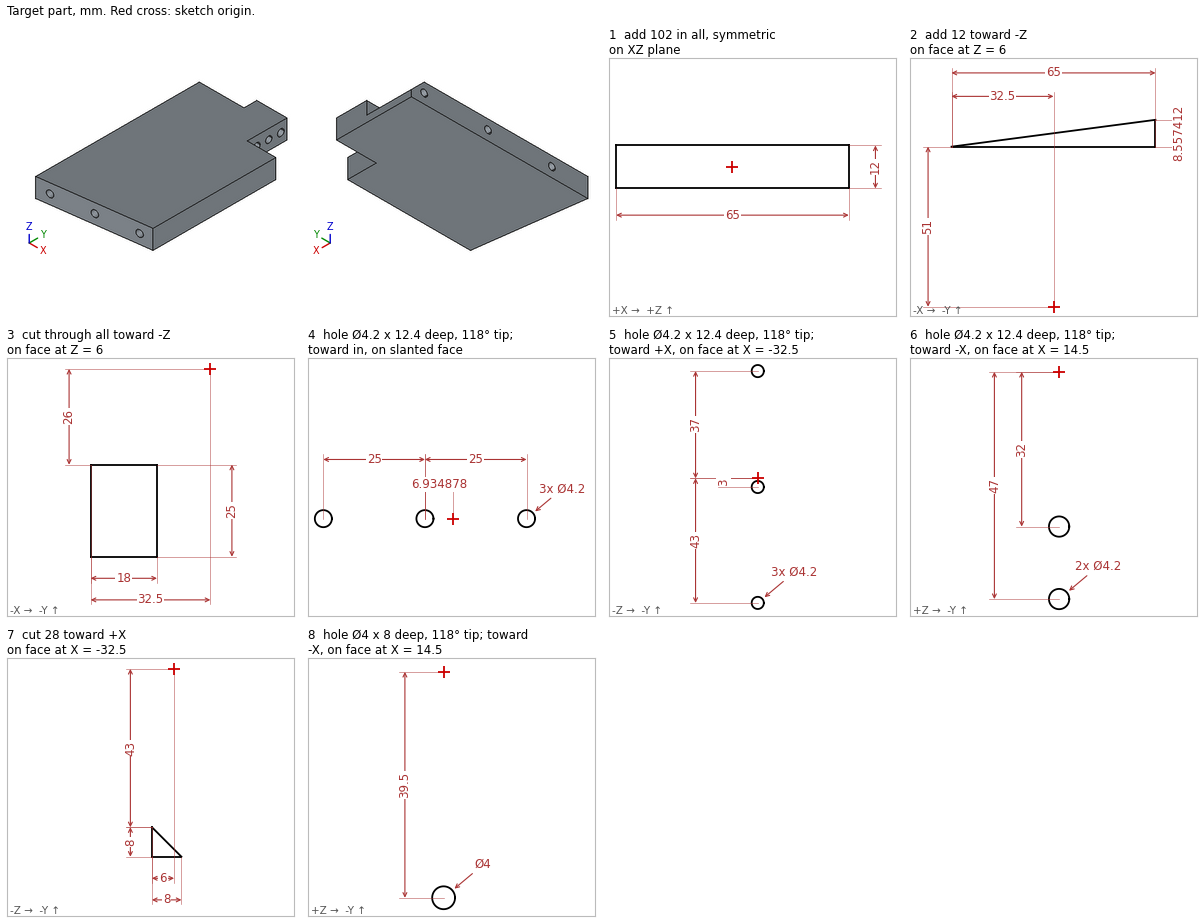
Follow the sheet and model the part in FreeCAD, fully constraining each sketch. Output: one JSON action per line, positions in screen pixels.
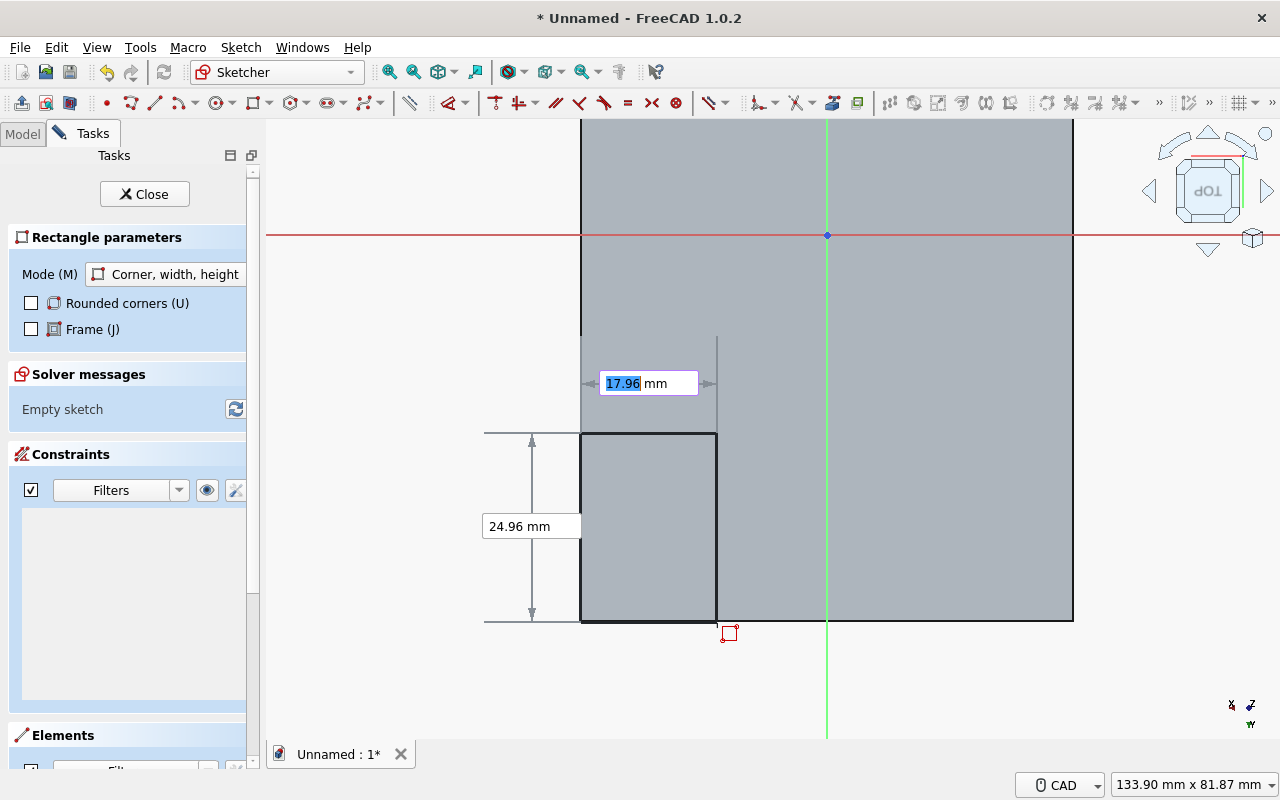
{"action": "type", "text": "18"}
{"action": "key", "text": "Tab"}
{"action": "type", "text": "25"}
{"action": "key", "text": "Return"}
{"action": "key", "text": "Escape"}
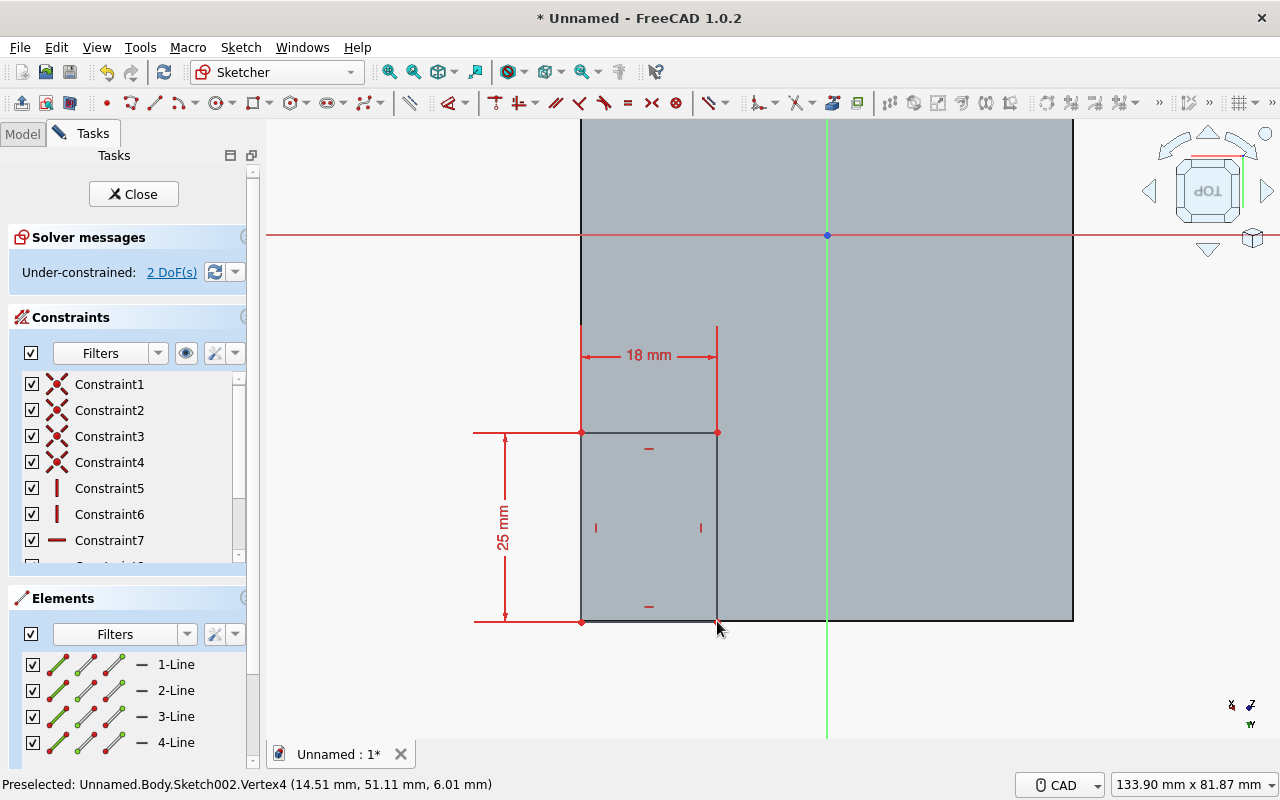
{"action": "left_click", "coordinate": [448, 104]}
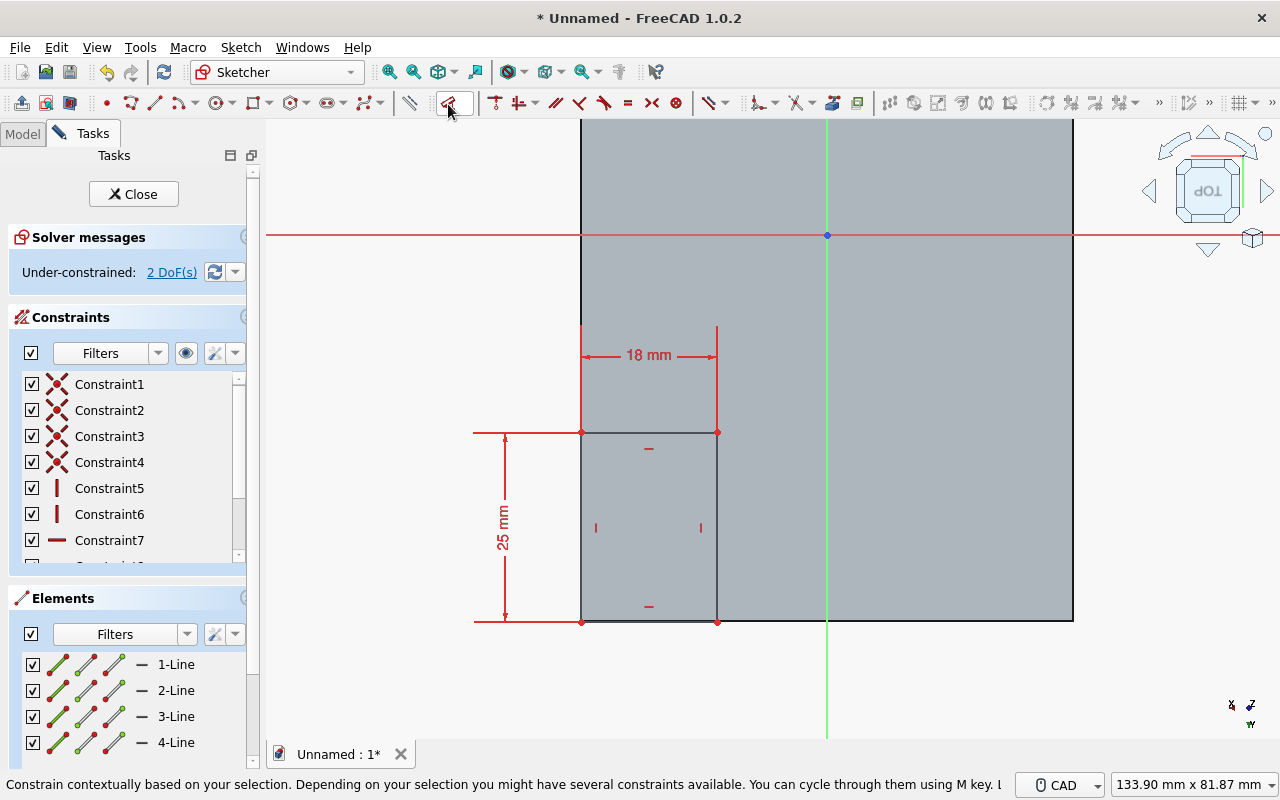
{"action": "left_click", "coordinate": [581, 433]}
{"action": "left_click", "coordinate": [547, 334]}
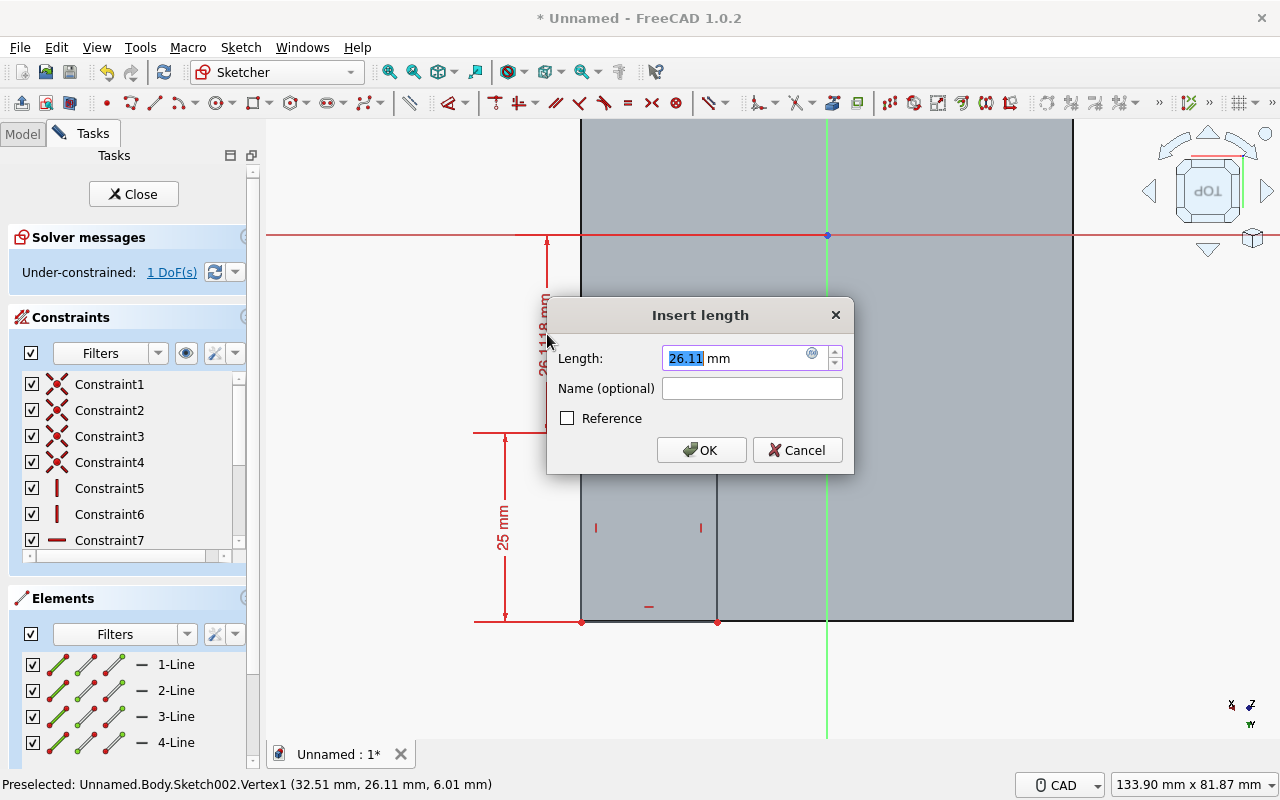
{"action": "type", "text": "26"}
{"action": "key", "text": "Return"}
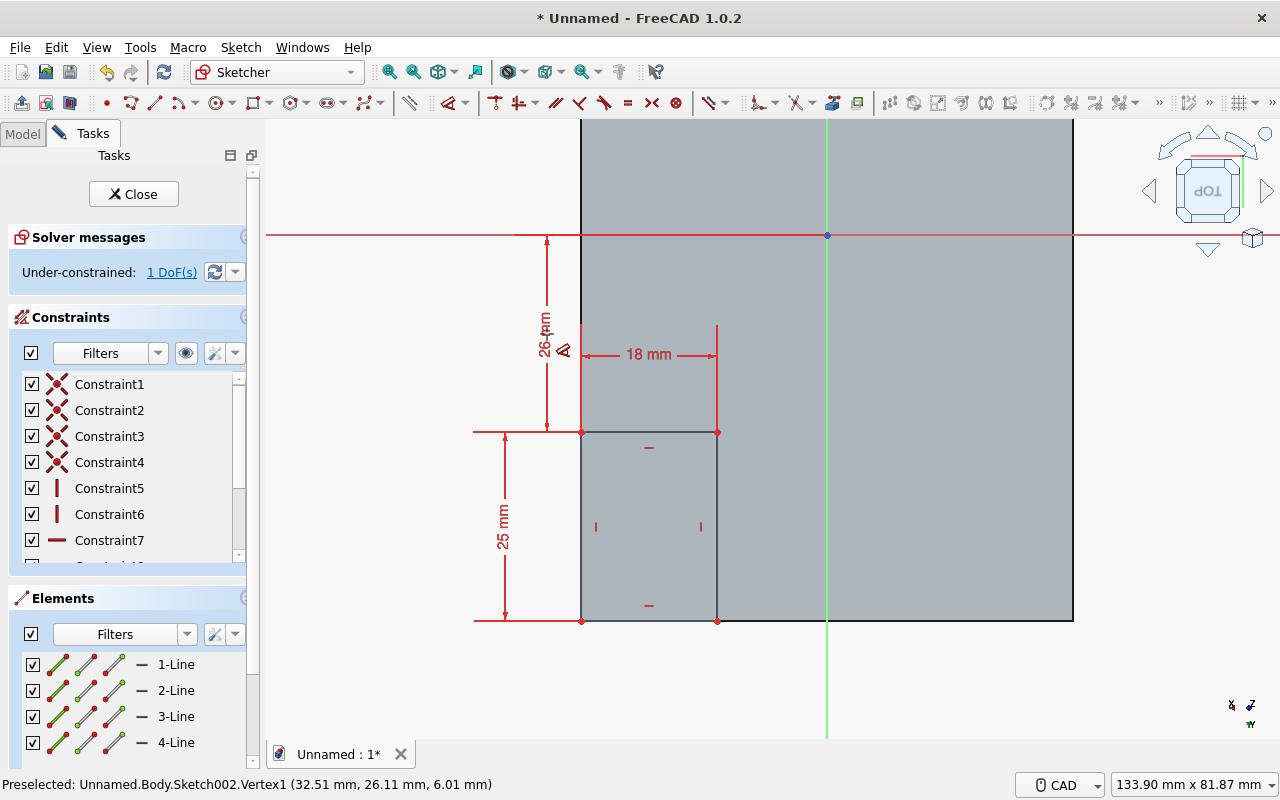
{"action": "left_click", "coordinate": [581, 432]}
{"action": "left_click", "coordinate": [704, 201]}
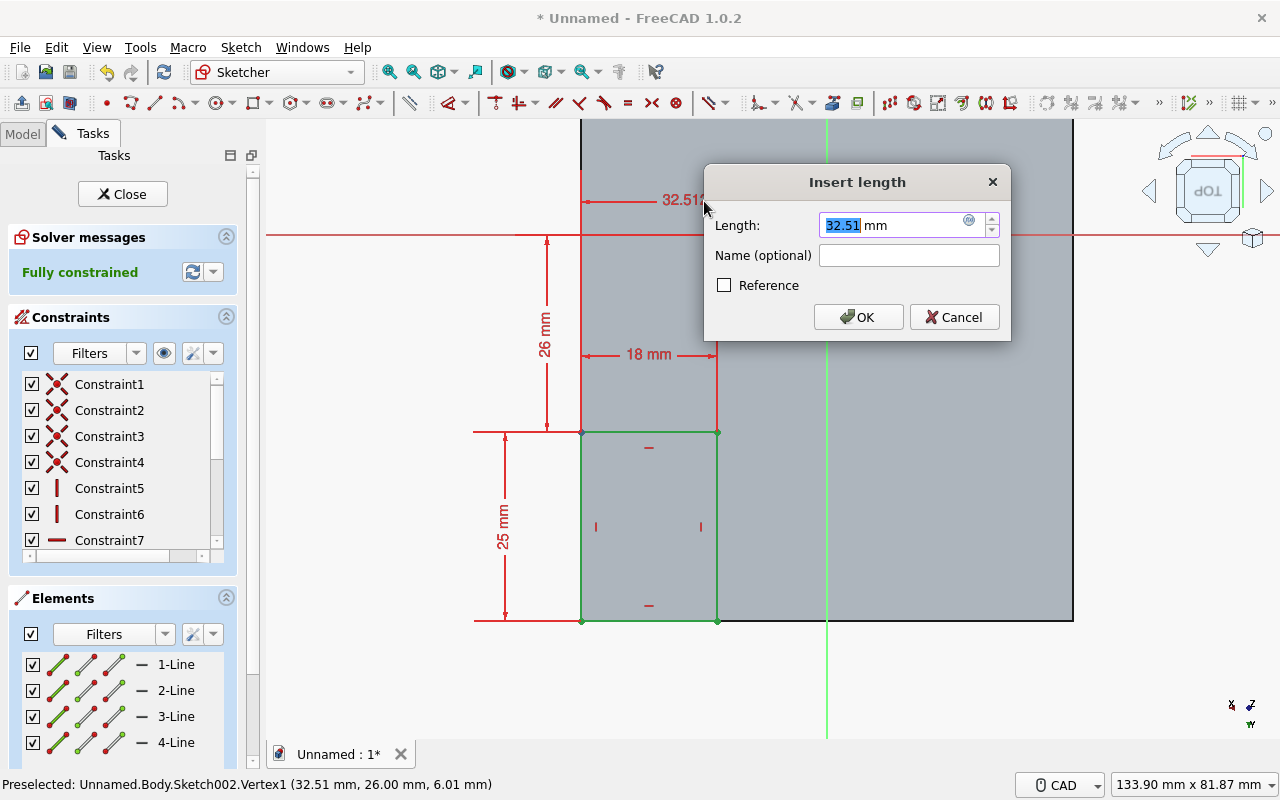
{"action": "type", "text": "32.5"}
{"action": "key", "text": "Return"}
{"action": "key", "text": "Escape"}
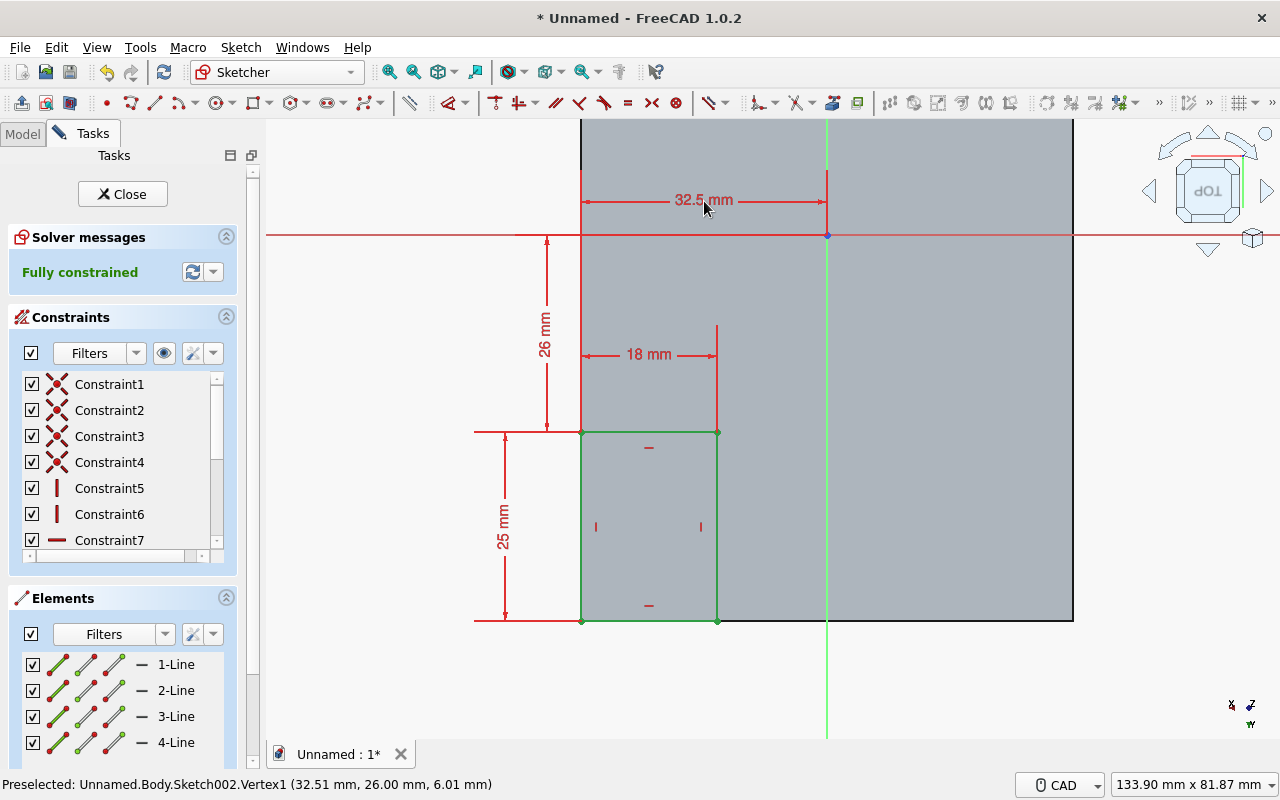
{"action": "left_click", "coordinate": [123, 194]}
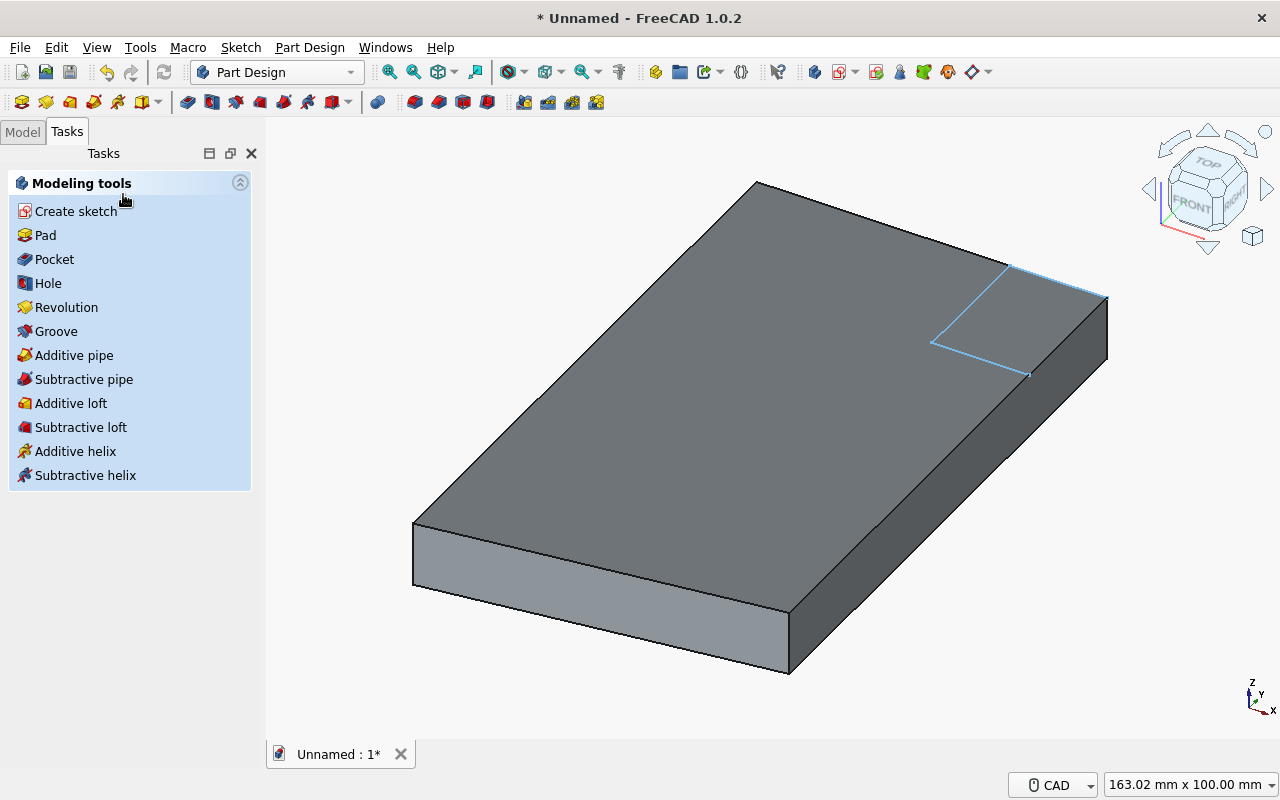
{"action": "left_click", "coordinate": [188, 102]}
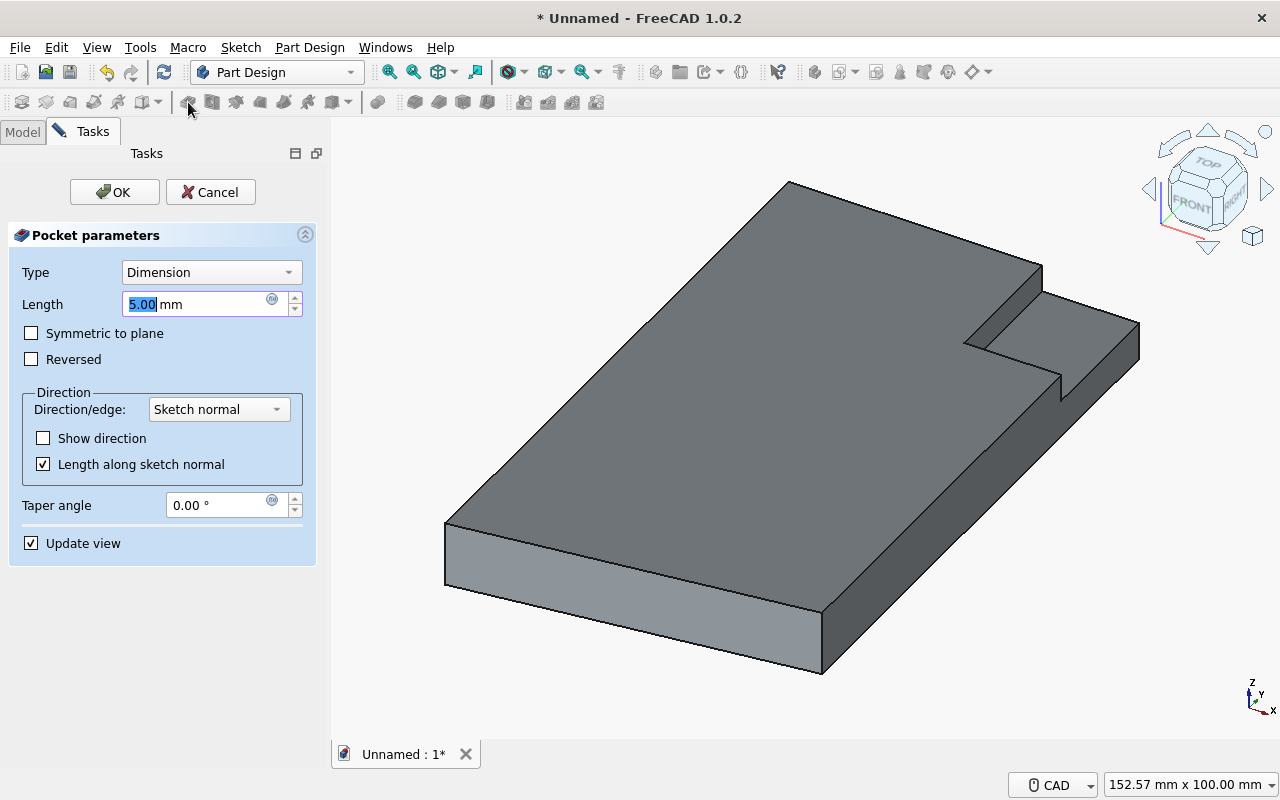
{"action": "left_click", "coordinate": [212, 272]}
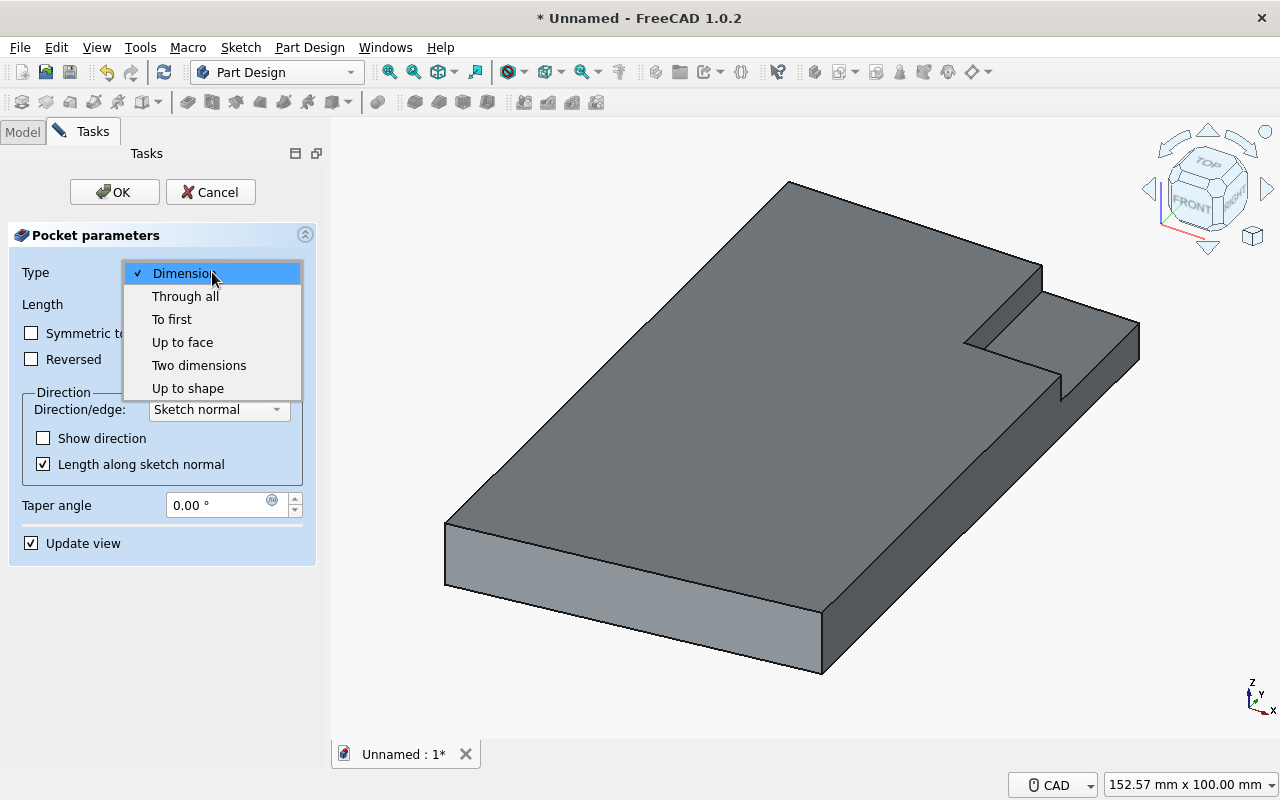
{"action": "left_click", "coordinate": [212, 296]}